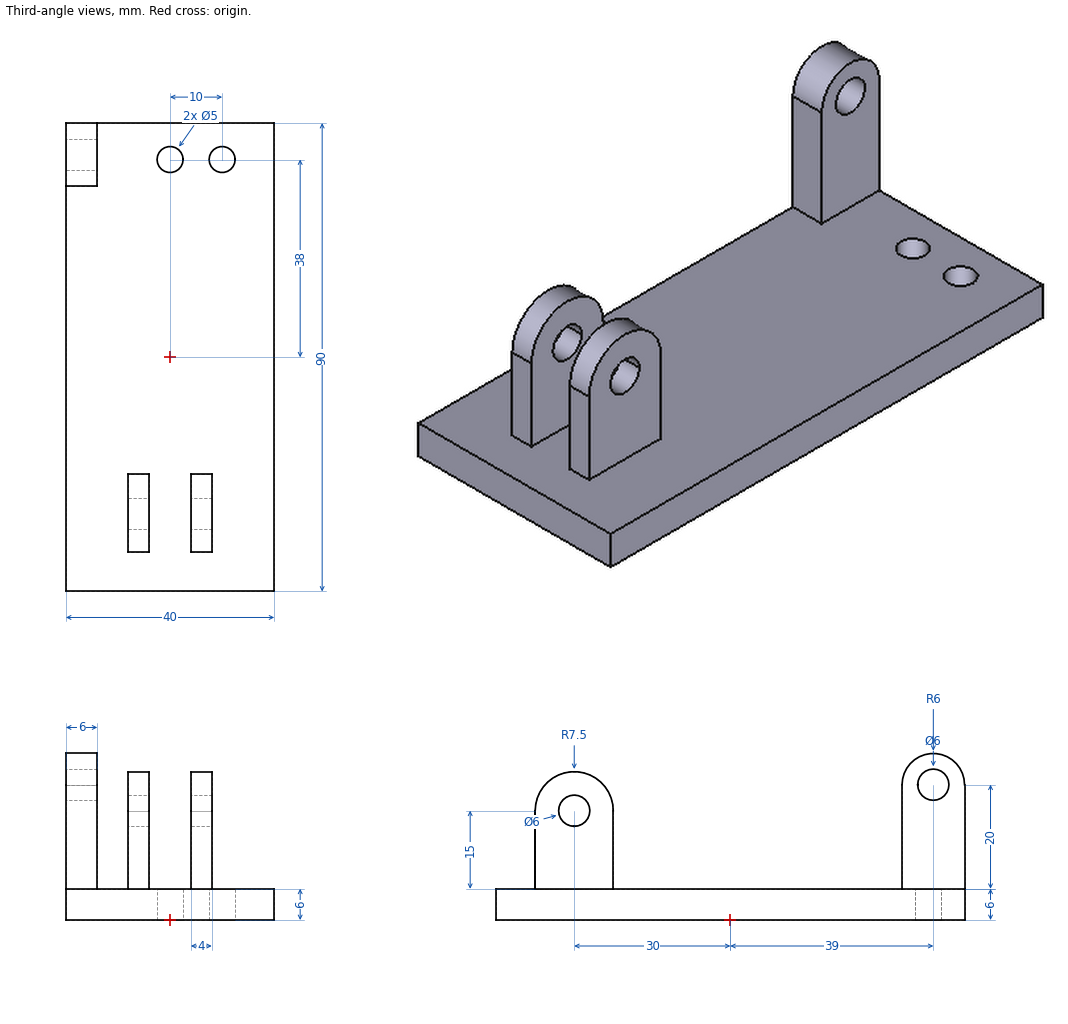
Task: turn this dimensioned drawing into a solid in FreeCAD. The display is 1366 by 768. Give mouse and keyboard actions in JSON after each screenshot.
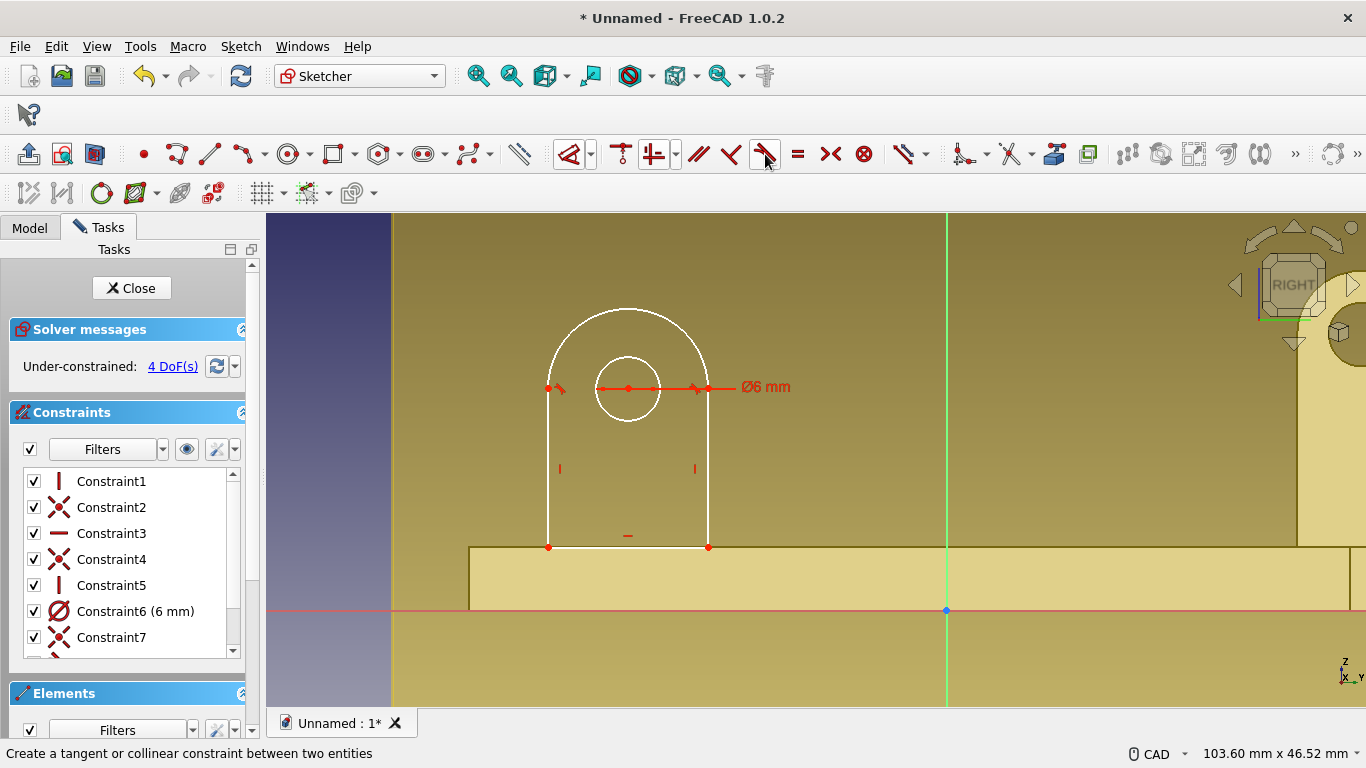
{"action": "key", "text": "d"}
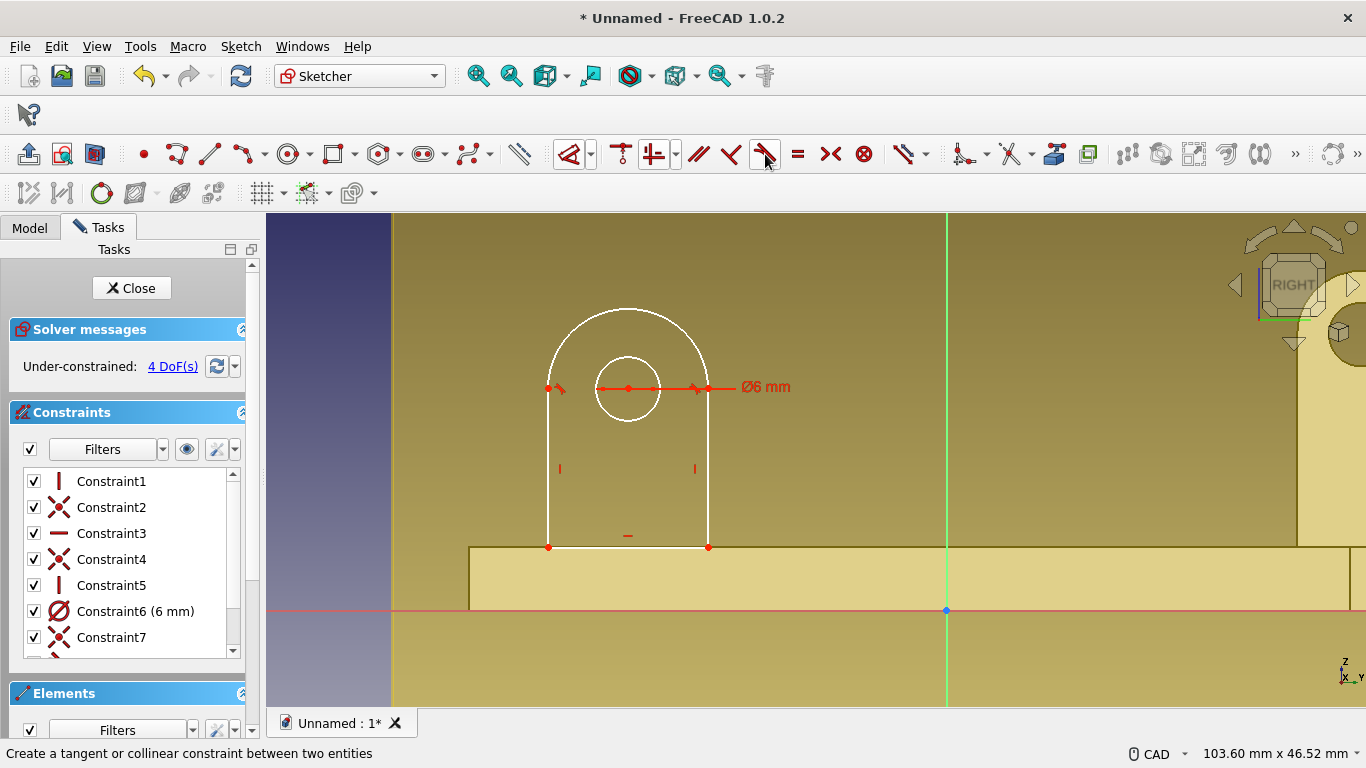
{"action": "left_click", "coordinate": [675, 324]}
{"action": "left_click", "coordinate": [694, 298]}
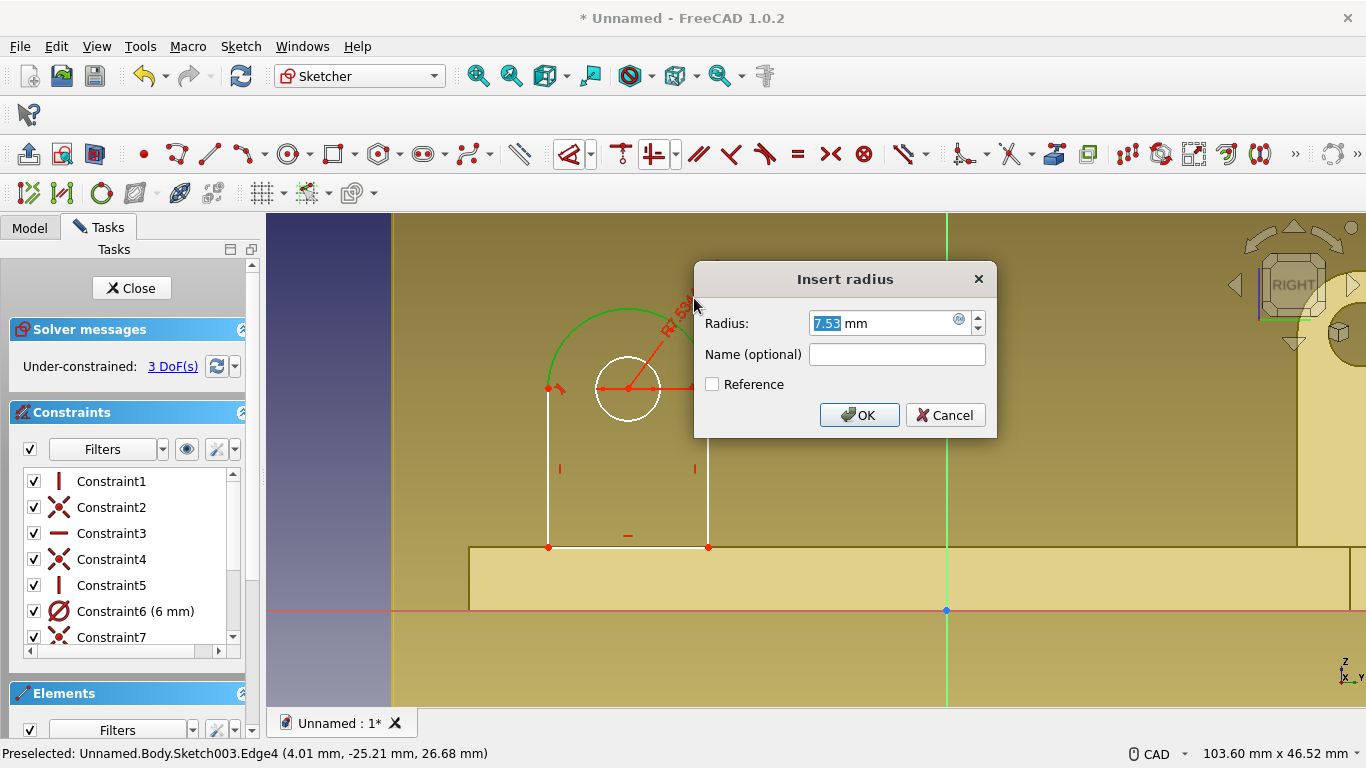
{"action": "type", "text": "7.5"}
{"action": "key", "text": "Return"}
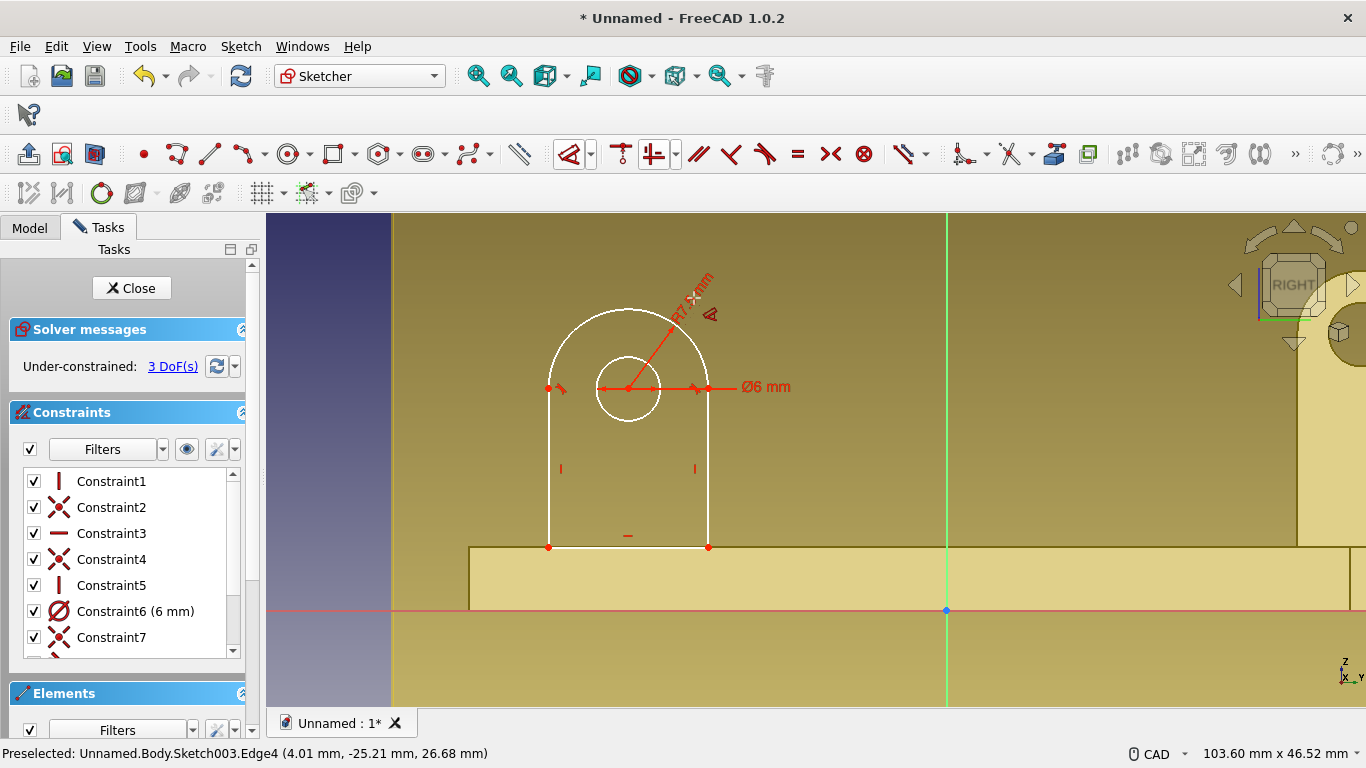
{"action": "left_click", "coordinate": [549, 437]}
{"action": "left_click", "coordinate": [515, 468]}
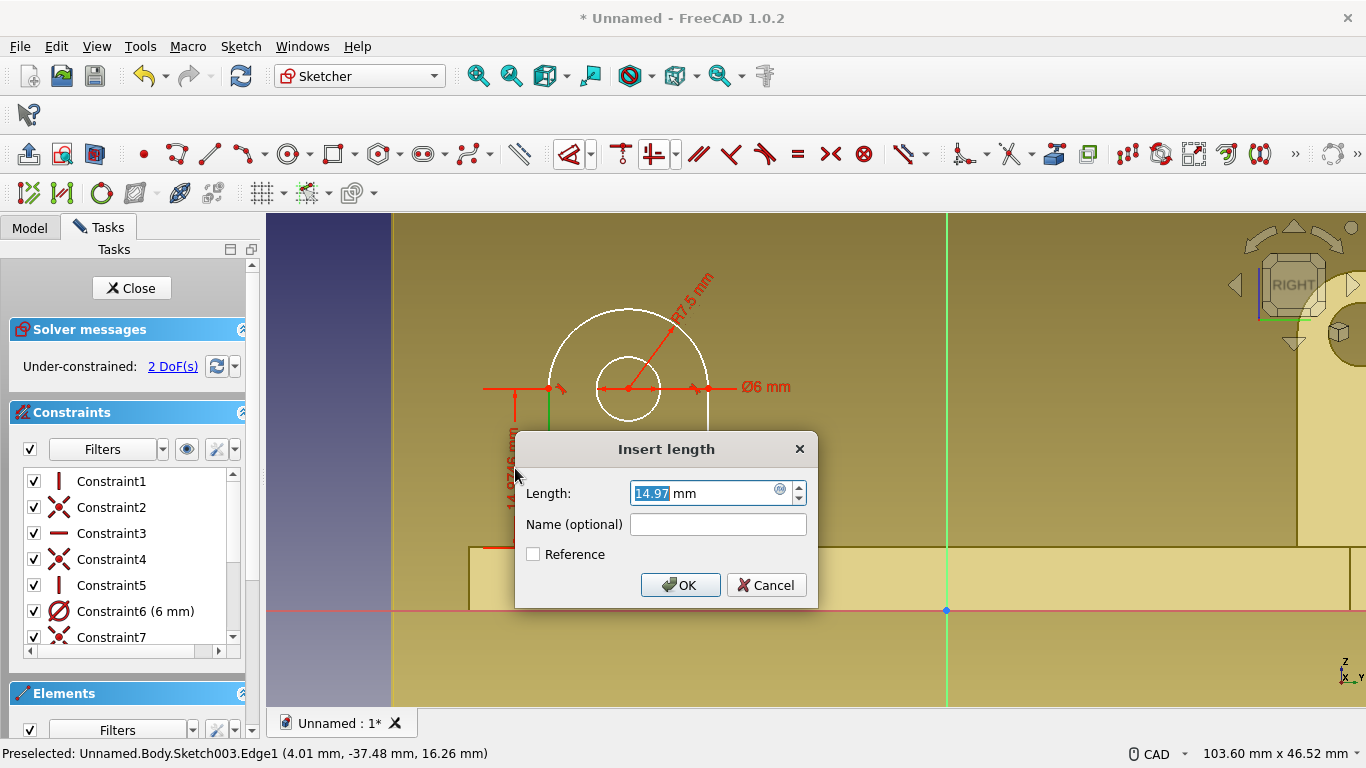
{"action": "type", "text": "15"}
{"action": "key", "text": "Return"}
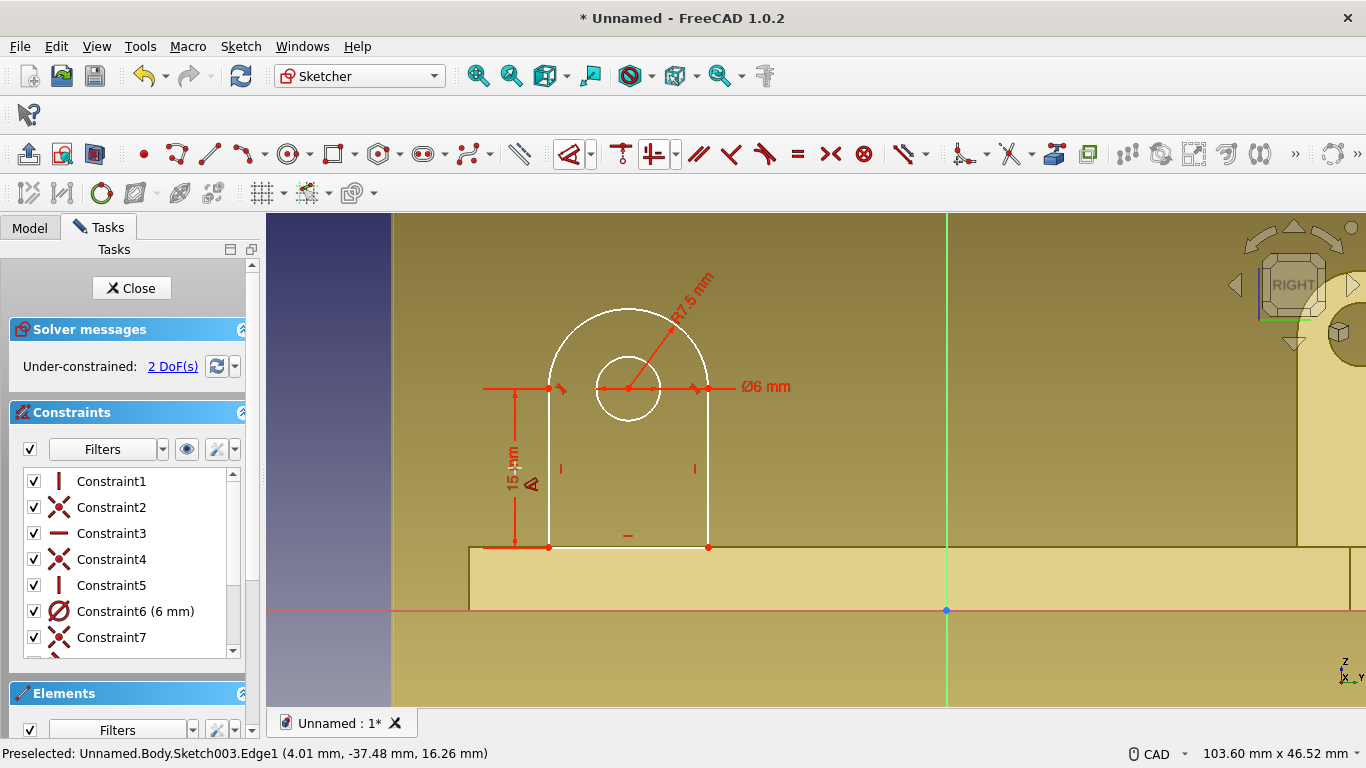
{"action": "left_click", "coordinate": [549, 548]}
{"action": "left_click", "coordinate": [981, 579]}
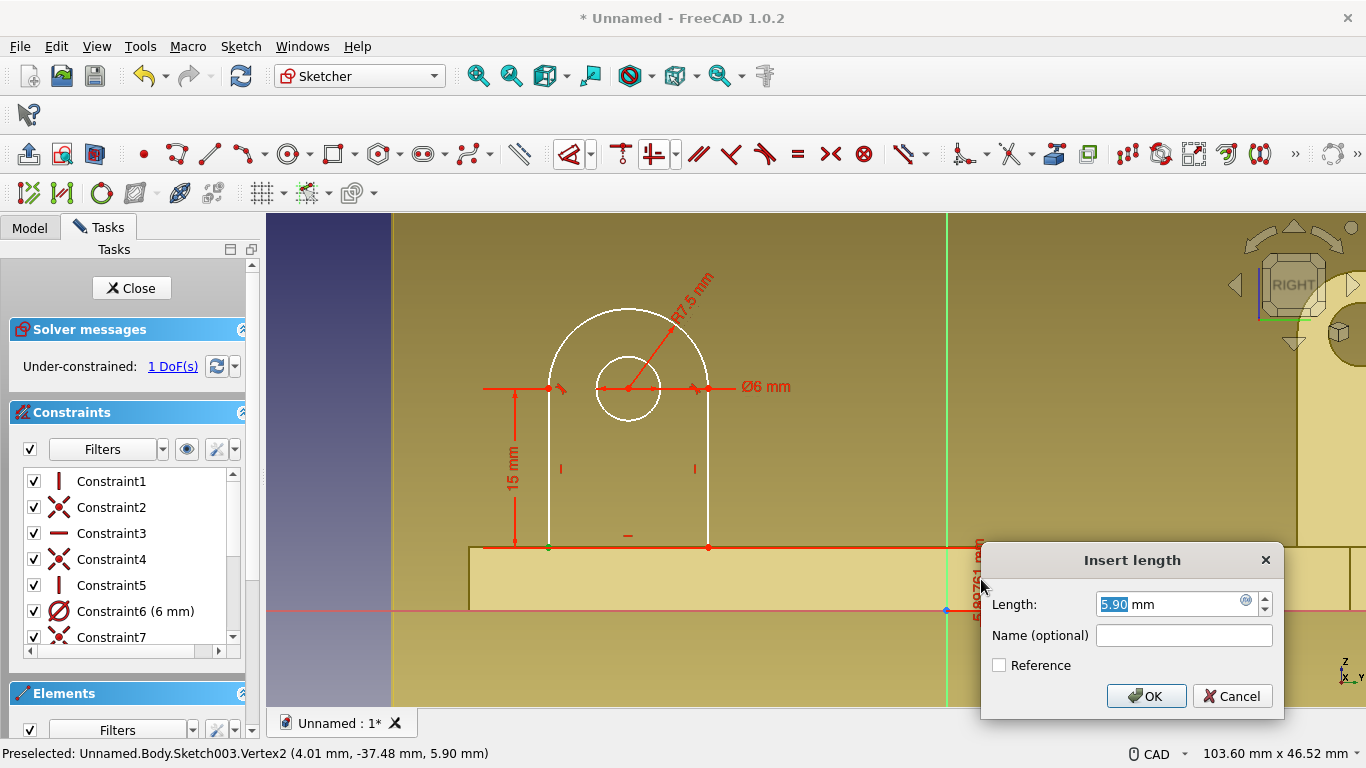
{"action": "type", "text": "6"}
{"action": "key", "text": "Return"}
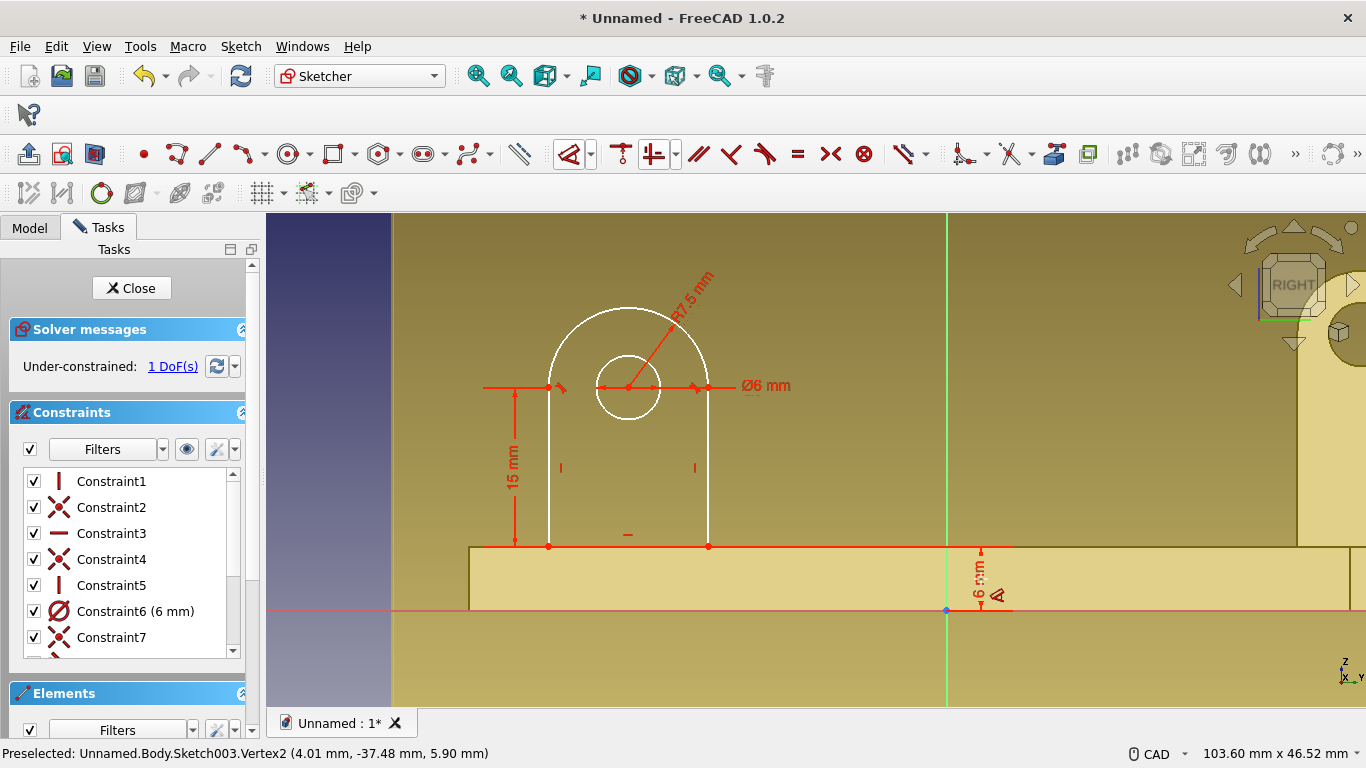
{"action": "left_click", "coordinate": [628, 388]}
{"action": "left_click", "coordinate": [788, 645]}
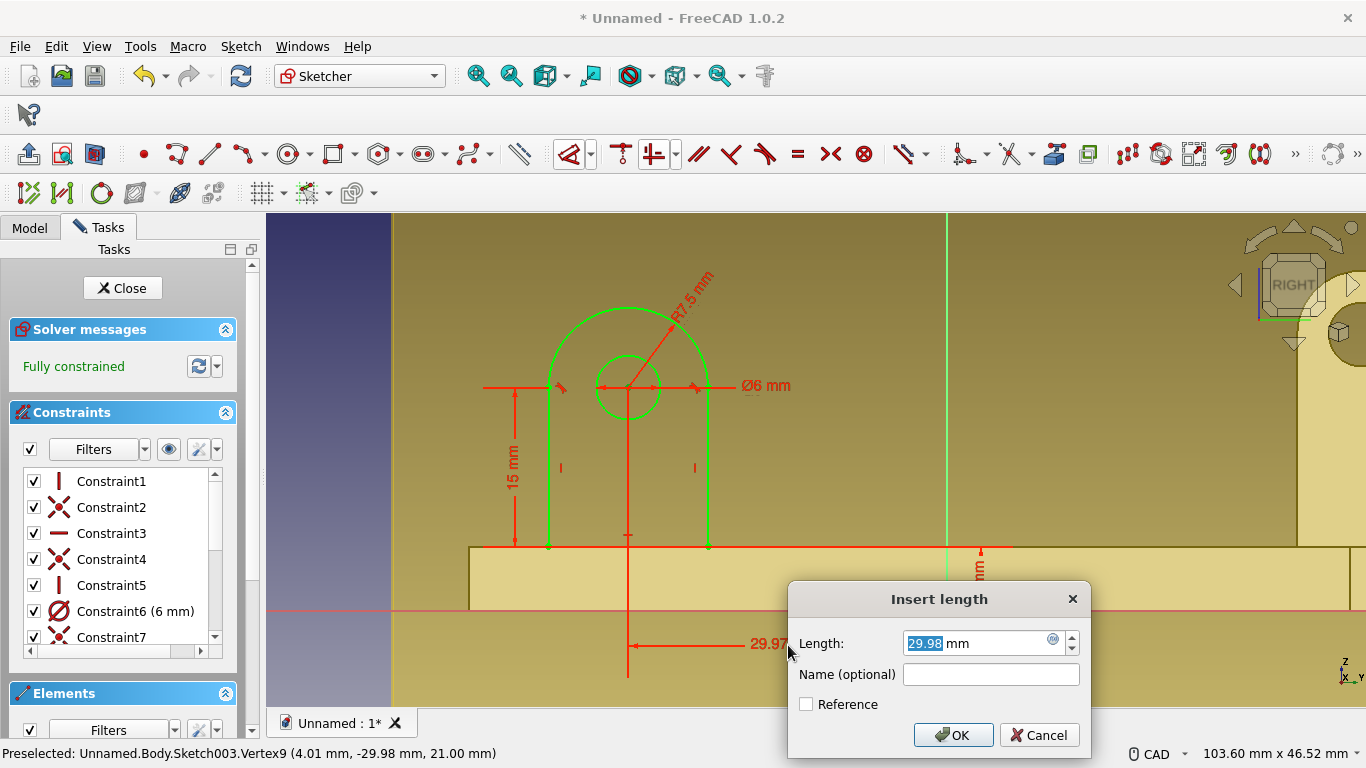
{"action": "type", "text": "30"}
{"action": "key", "text": "Return"}
{"action": "key", "text": "Escape"}